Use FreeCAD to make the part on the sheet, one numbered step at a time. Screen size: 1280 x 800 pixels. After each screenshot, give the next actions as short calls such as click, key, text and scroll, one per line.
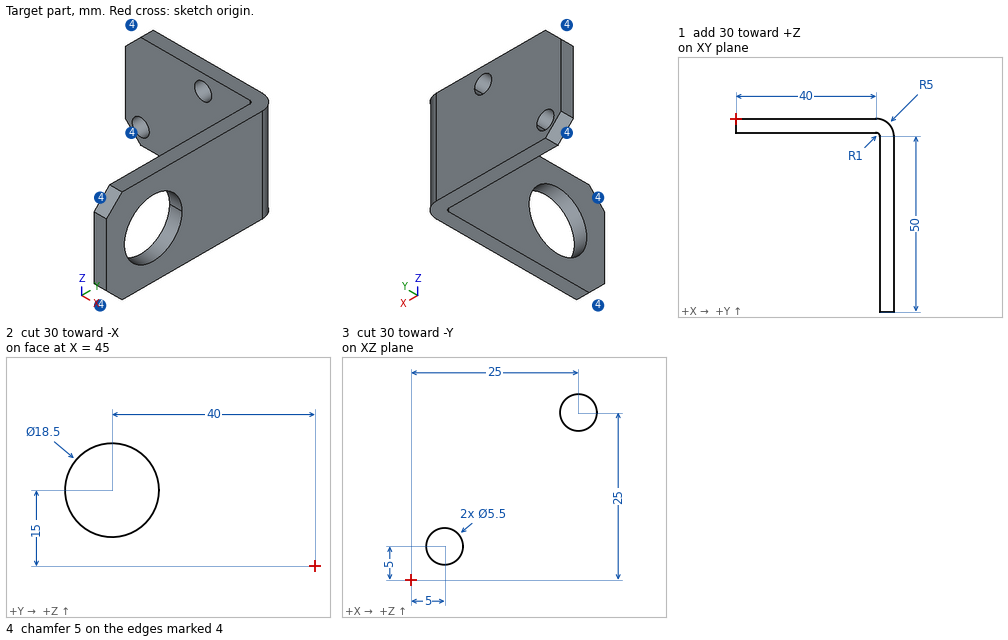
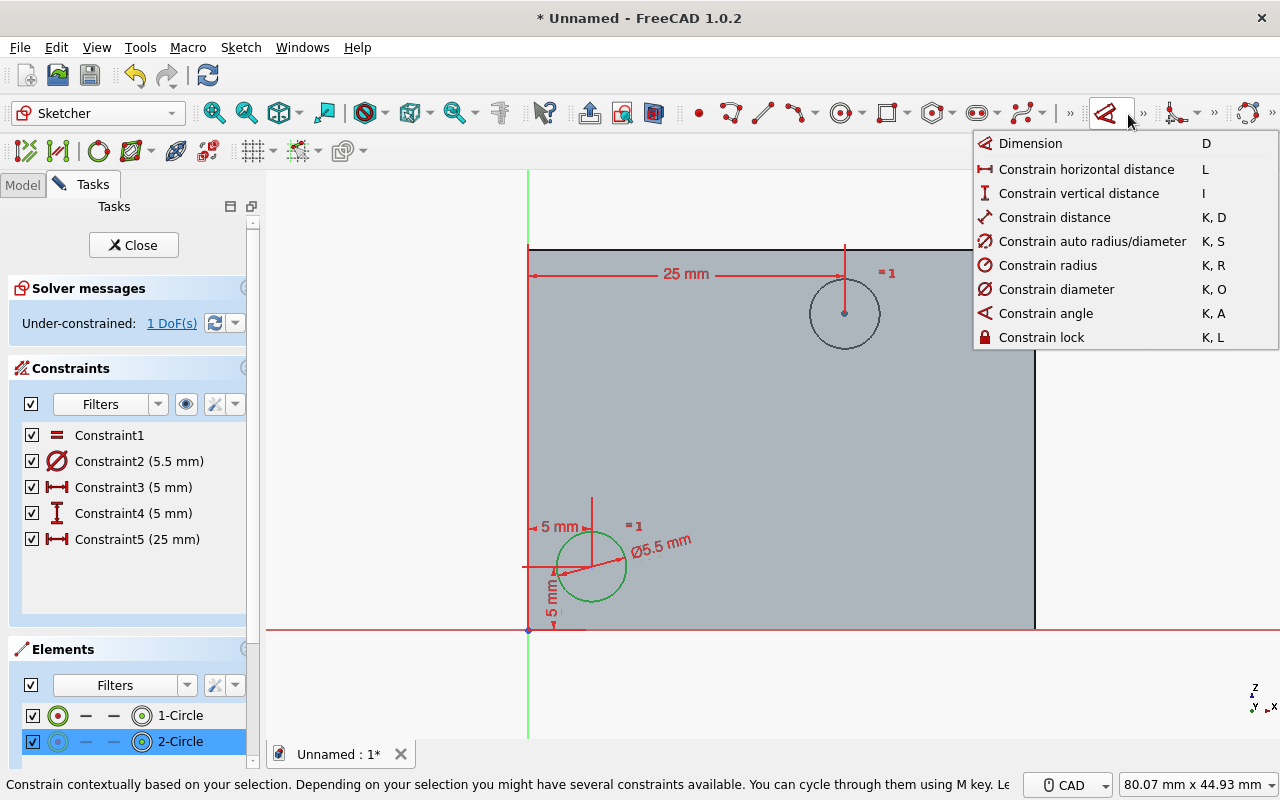
click(1126, 193)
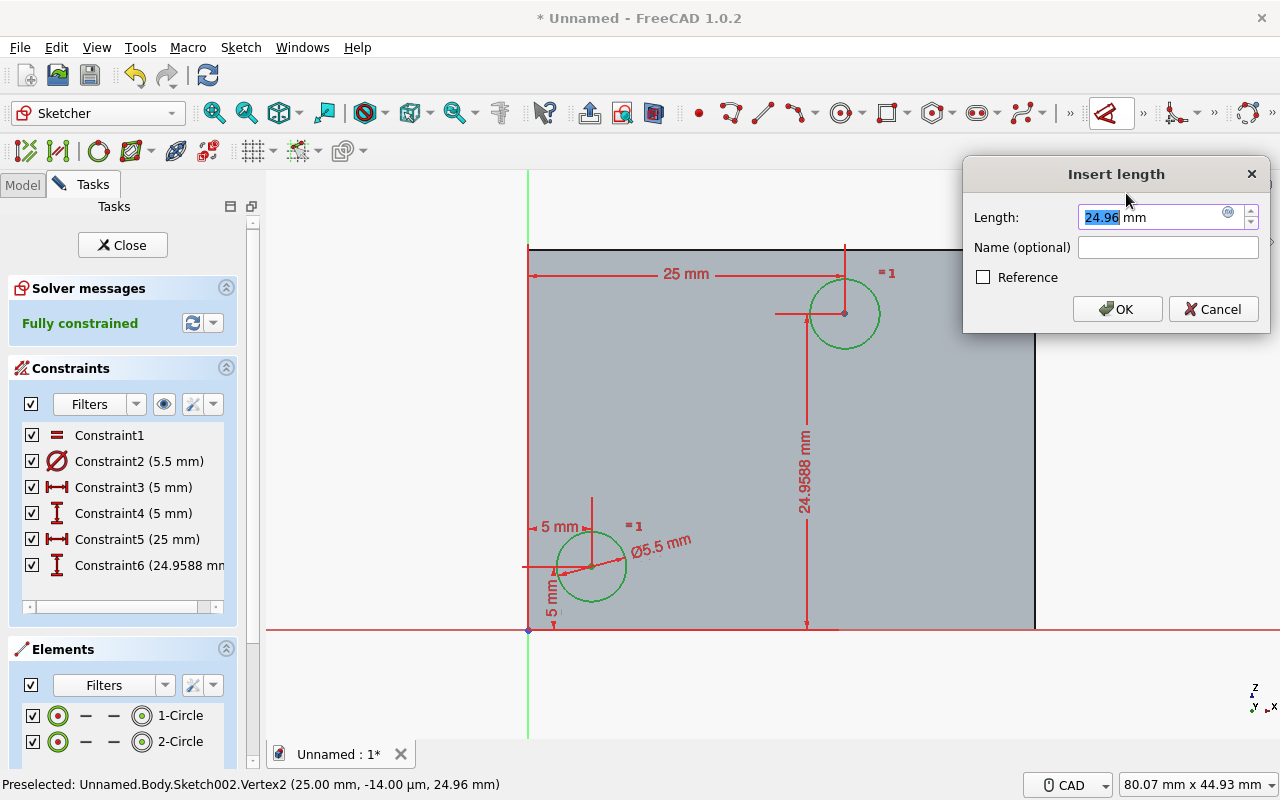
text(25)
key(Return)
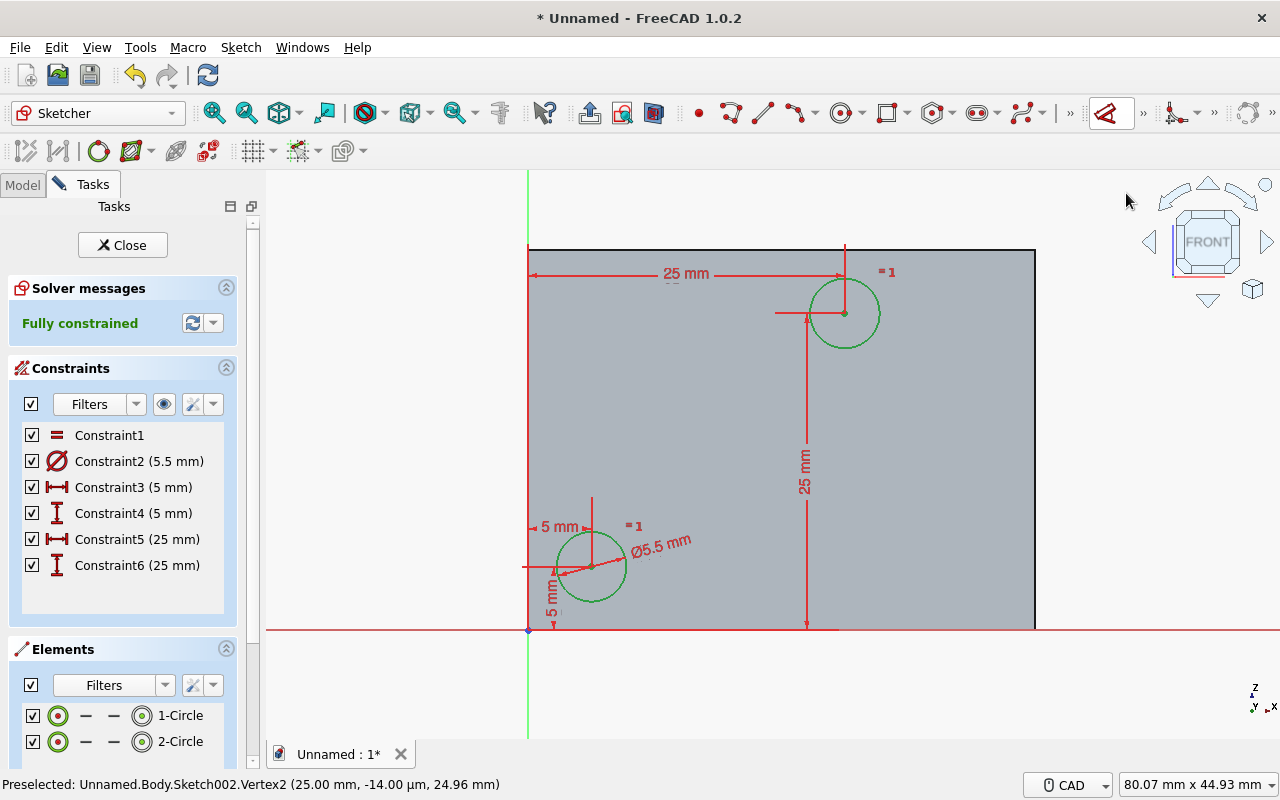
click(123, 245)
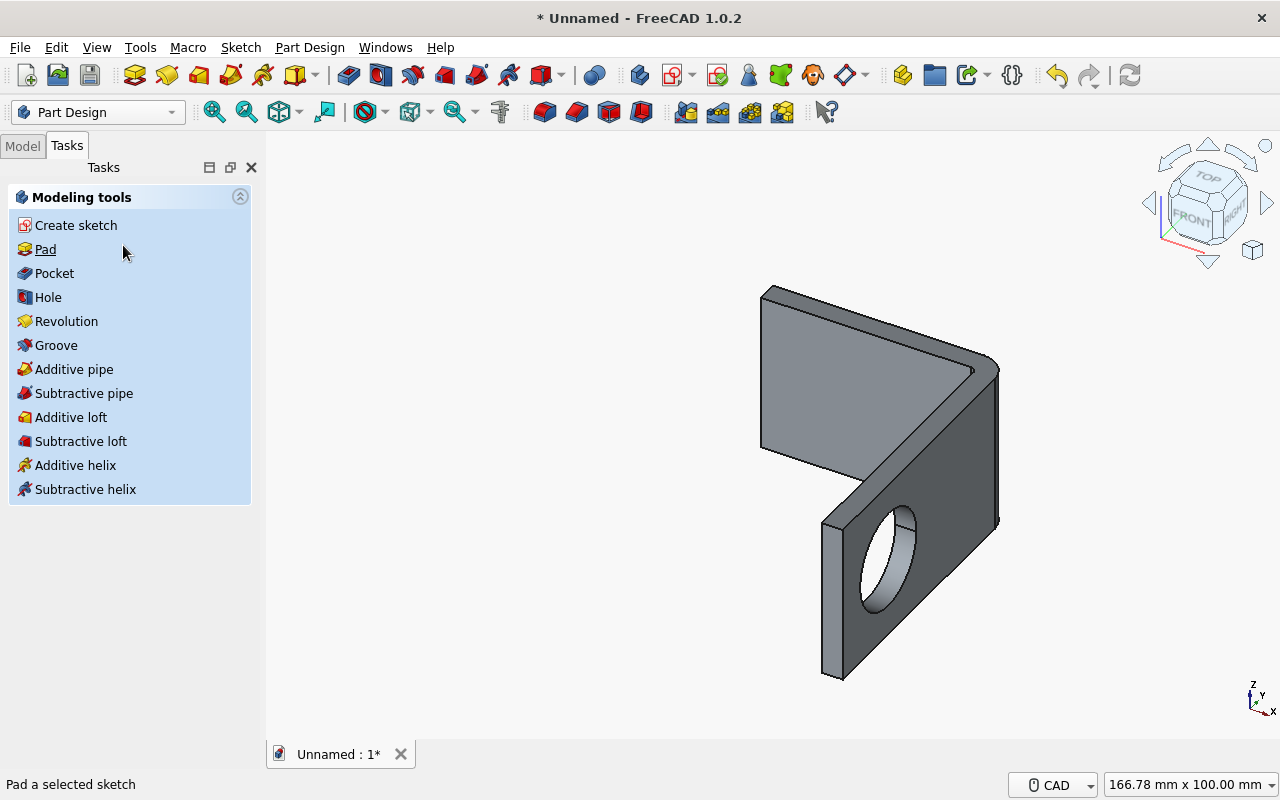
click(350, 76)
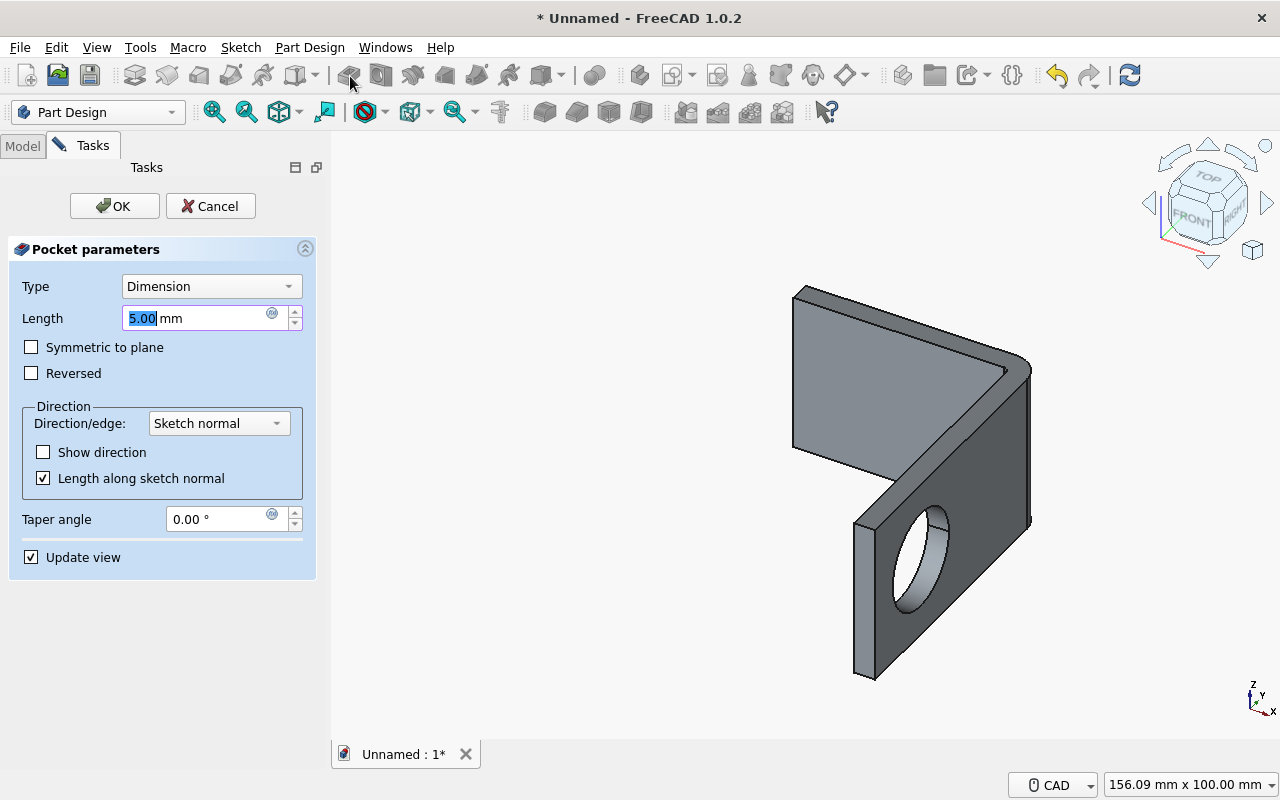
text(30)
key(Tab)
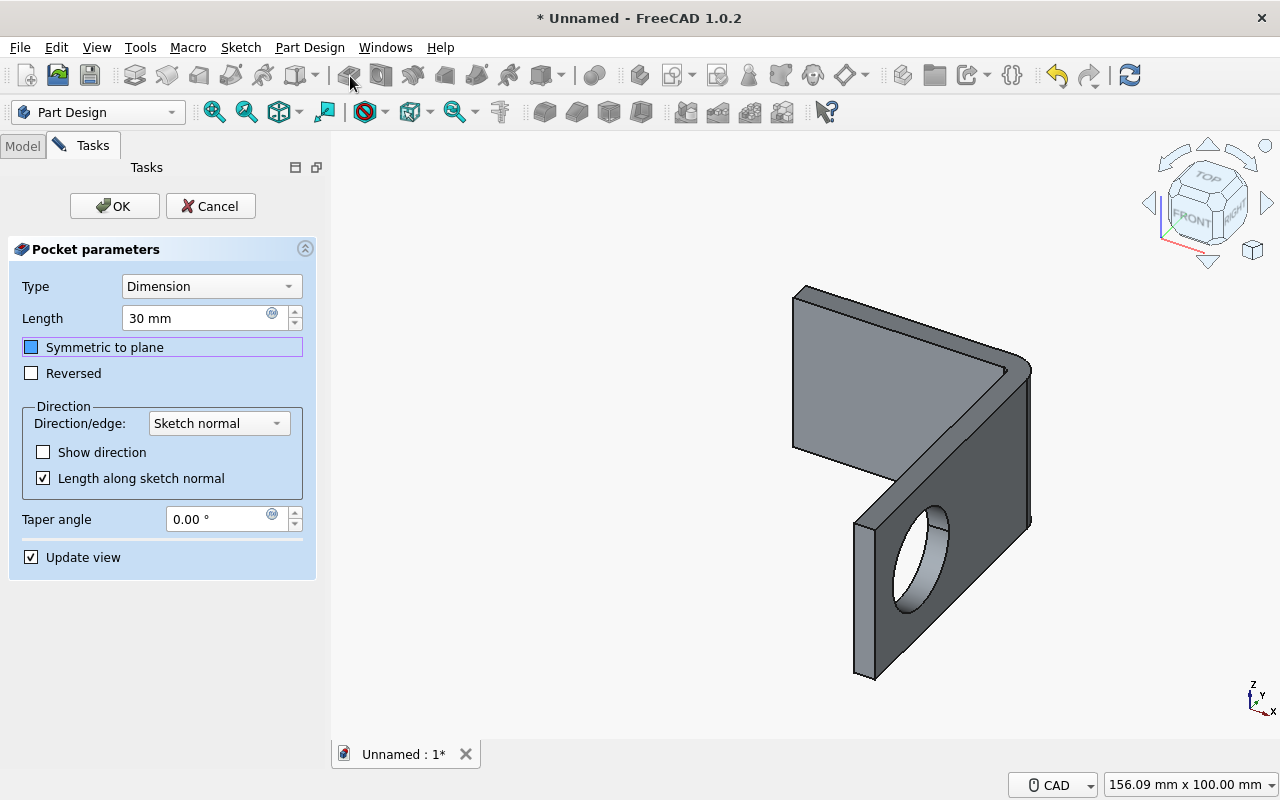
click(30, 373)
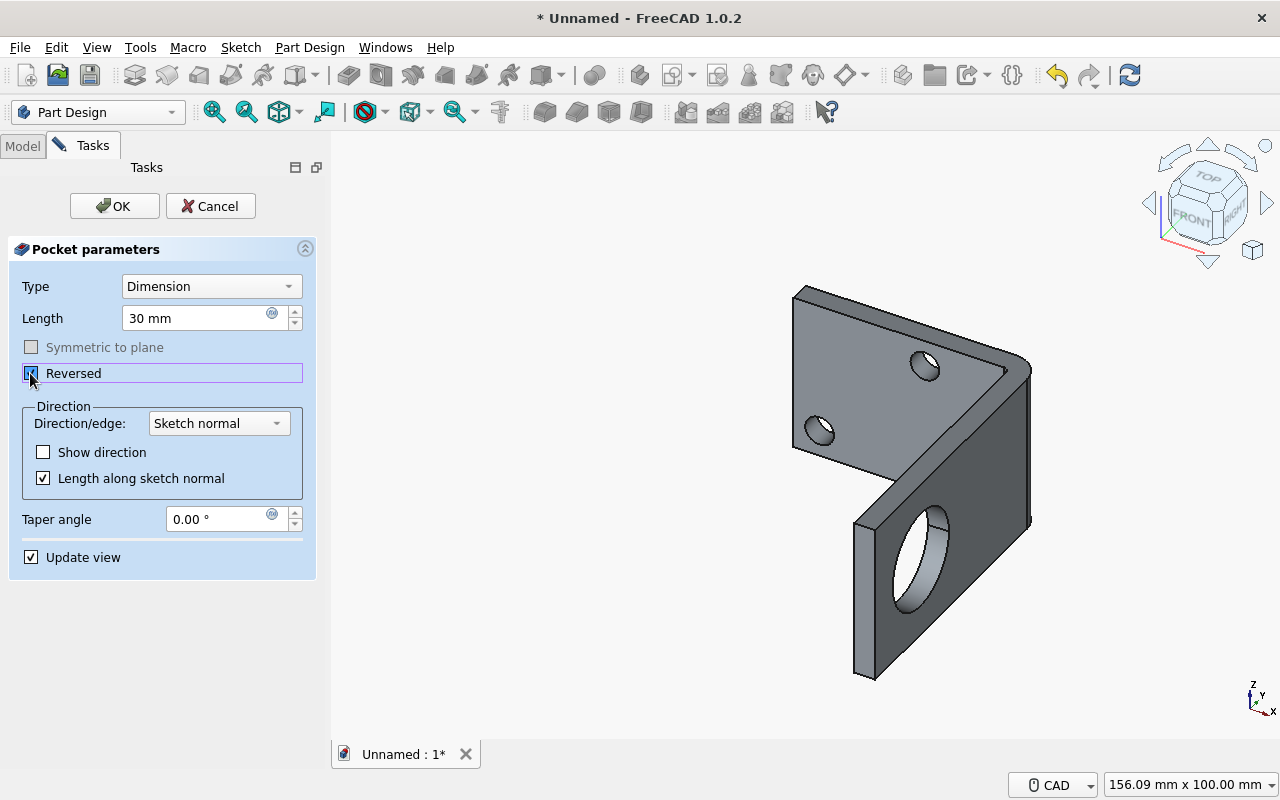
click(115, 206)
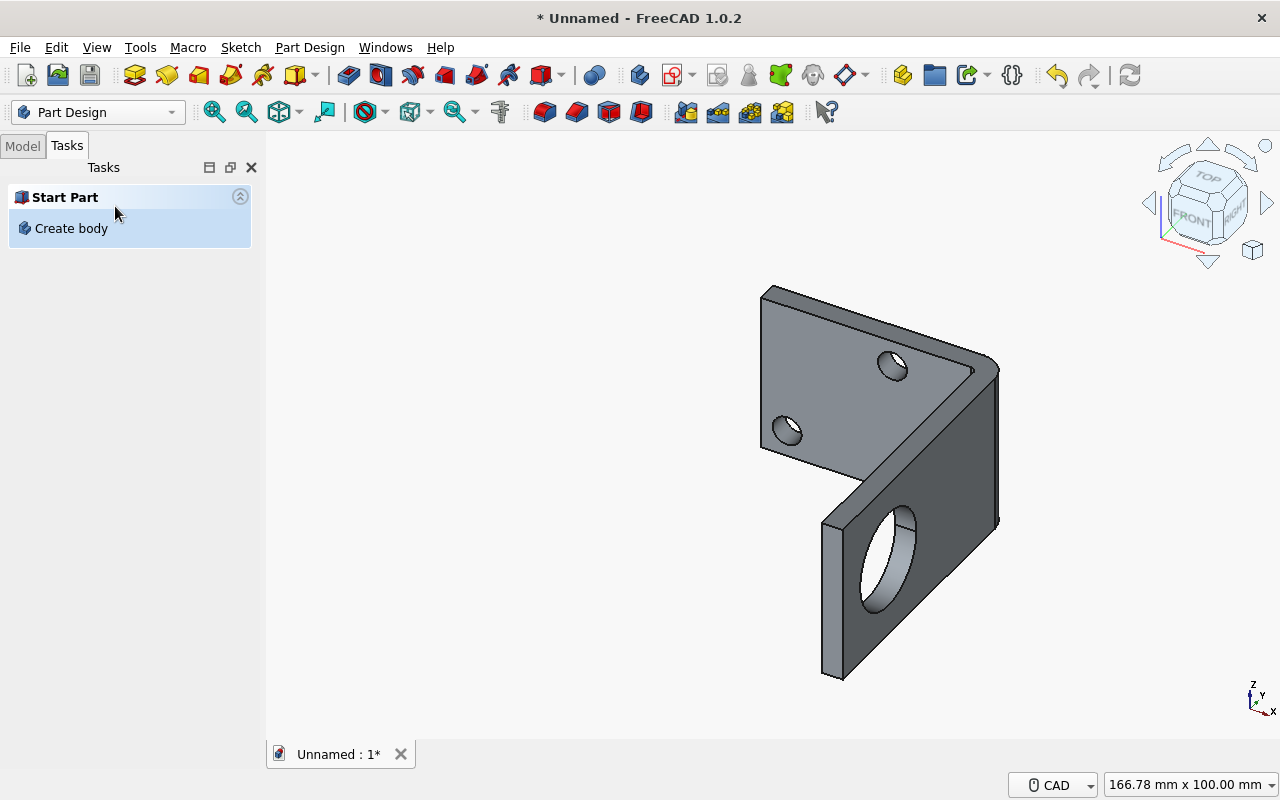
click(832, 526)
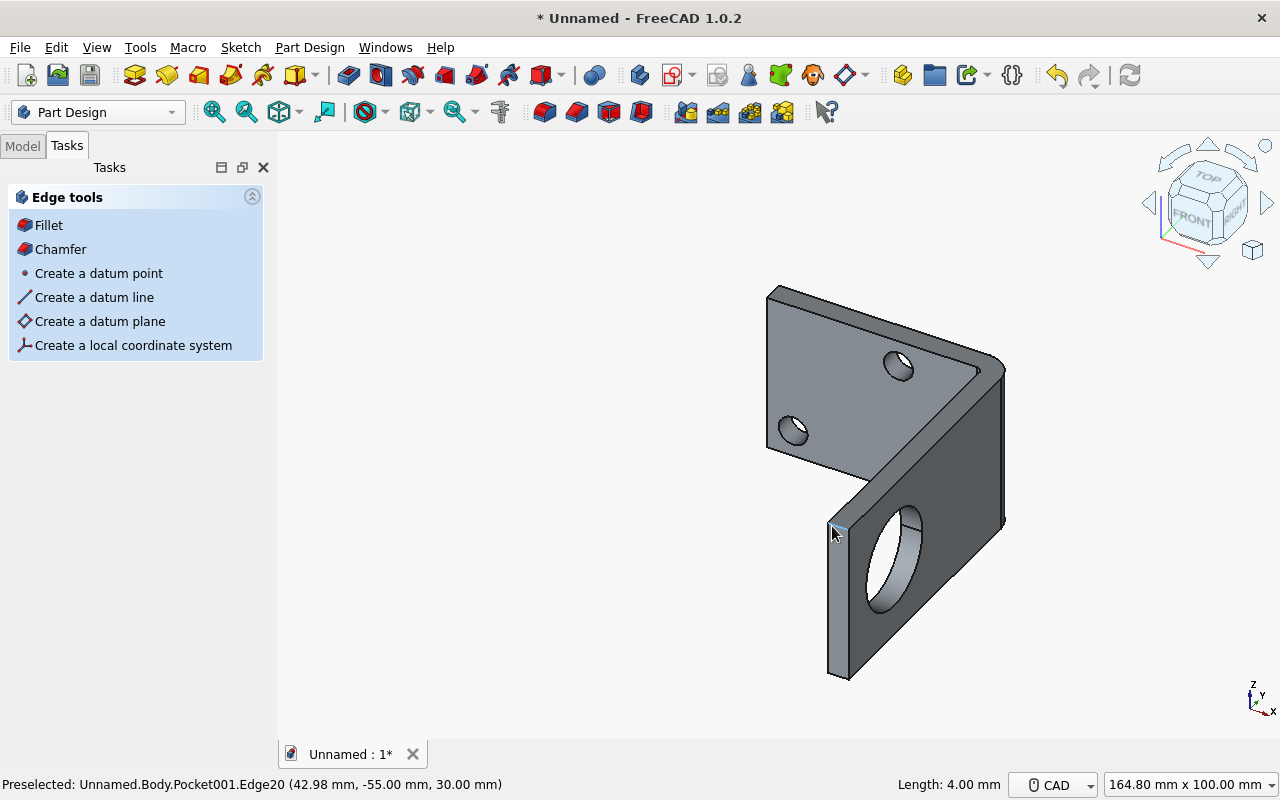
key(0)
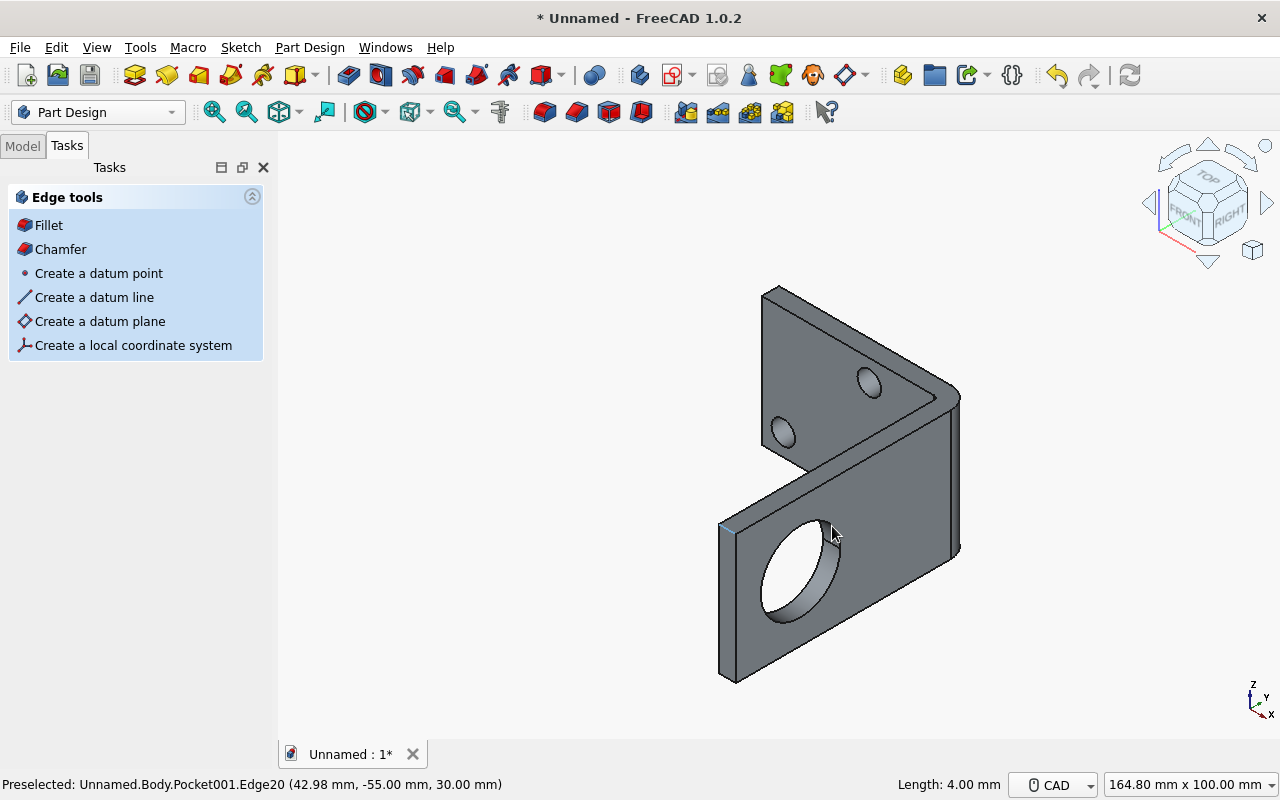
key(2)